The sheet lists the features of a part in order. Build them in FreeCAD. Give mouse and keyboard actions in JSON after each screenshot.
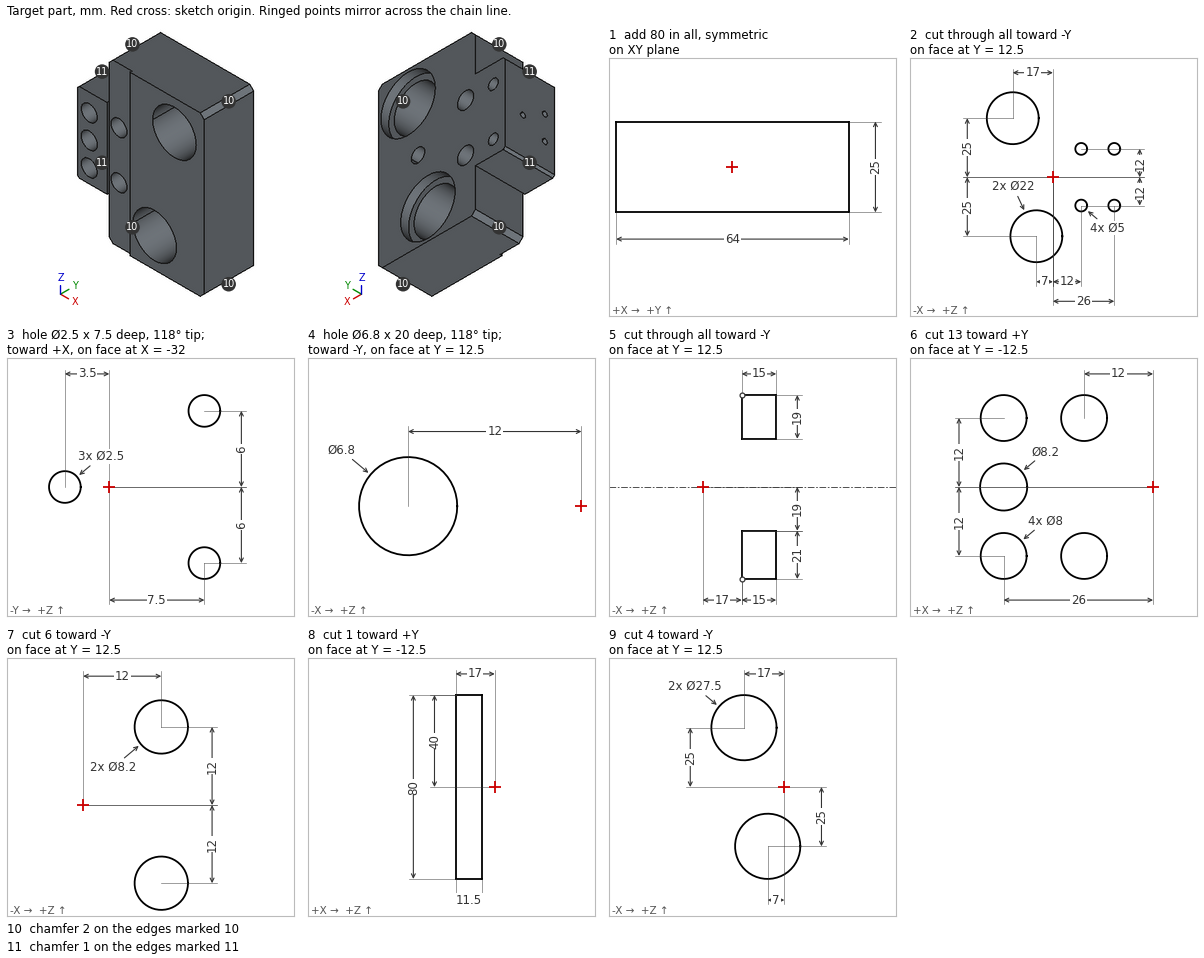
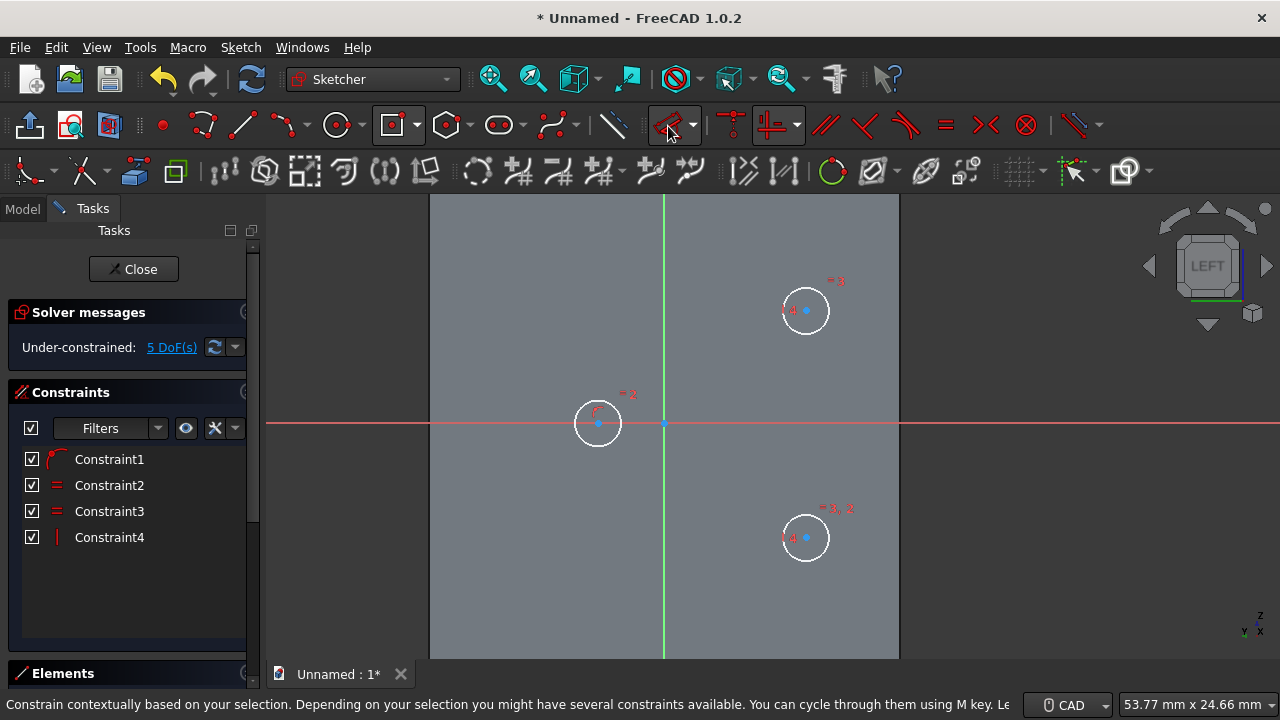
{"action": "left_click", "coordinate": [614, 407]}
{"action": "left_click", "coordinate": [636, 384]}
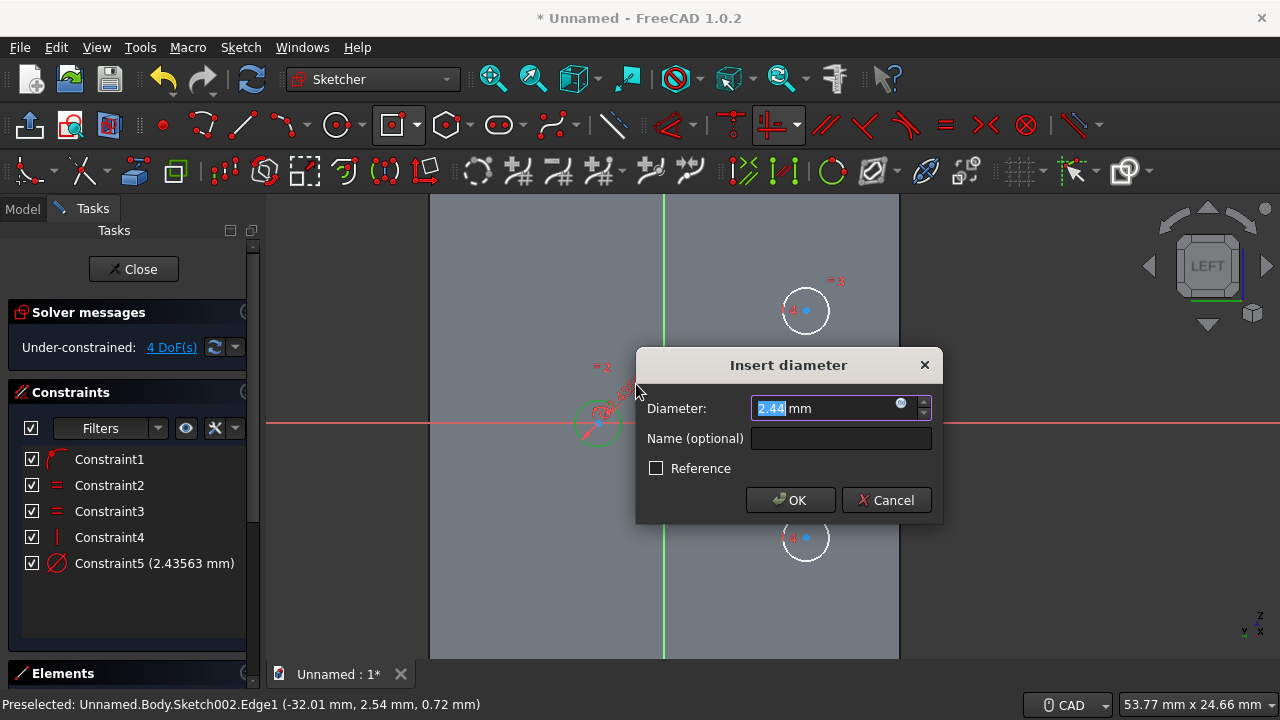
{"action": "type", "text": "2.5"}
{"action": "key", "text": "Return"}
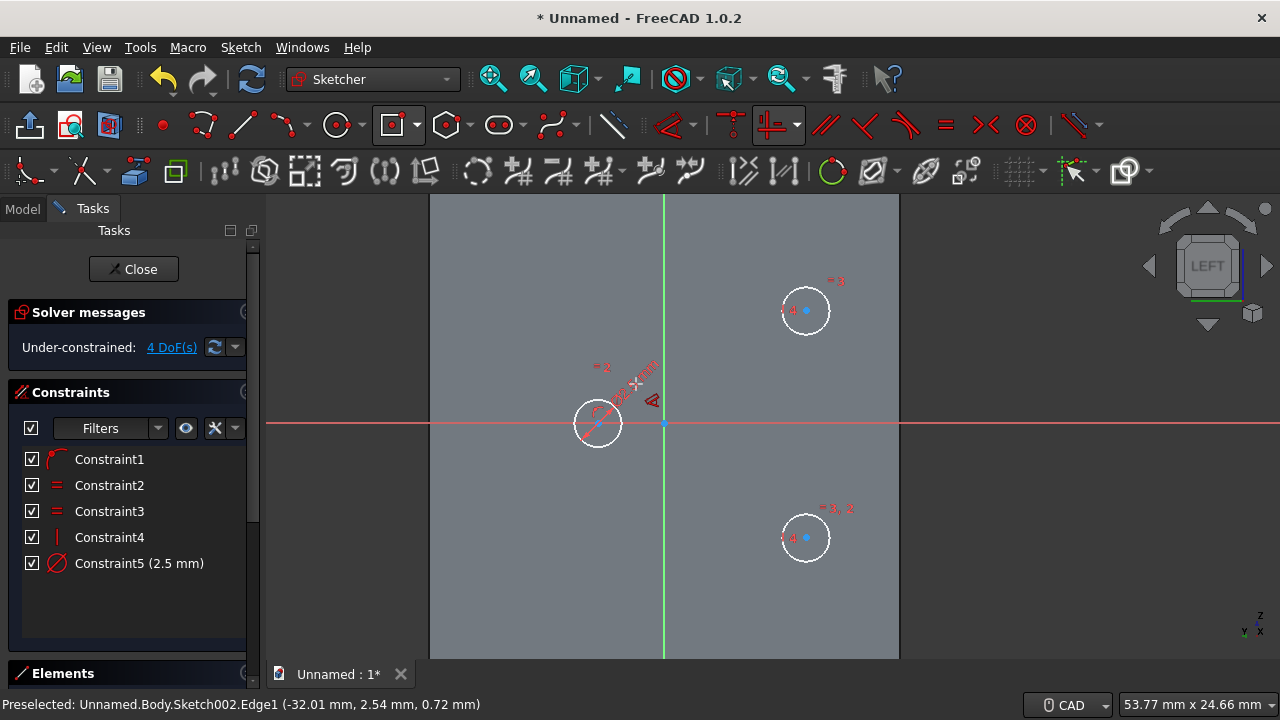
{"action": "left_click", "coordinate": [806, 538]}
{"action": "left_click", "coordinate": [840, 481]}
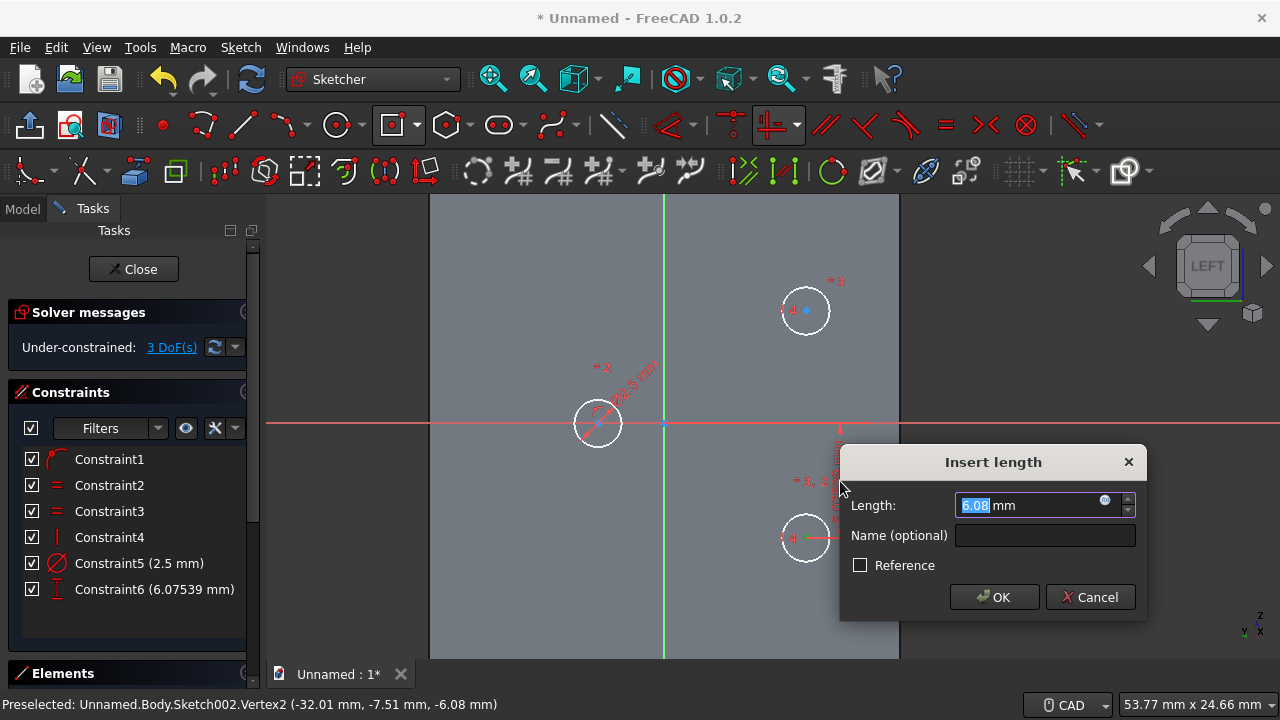
{"action": "type", "text": "6"}
{"action": "key", "text": "Return"}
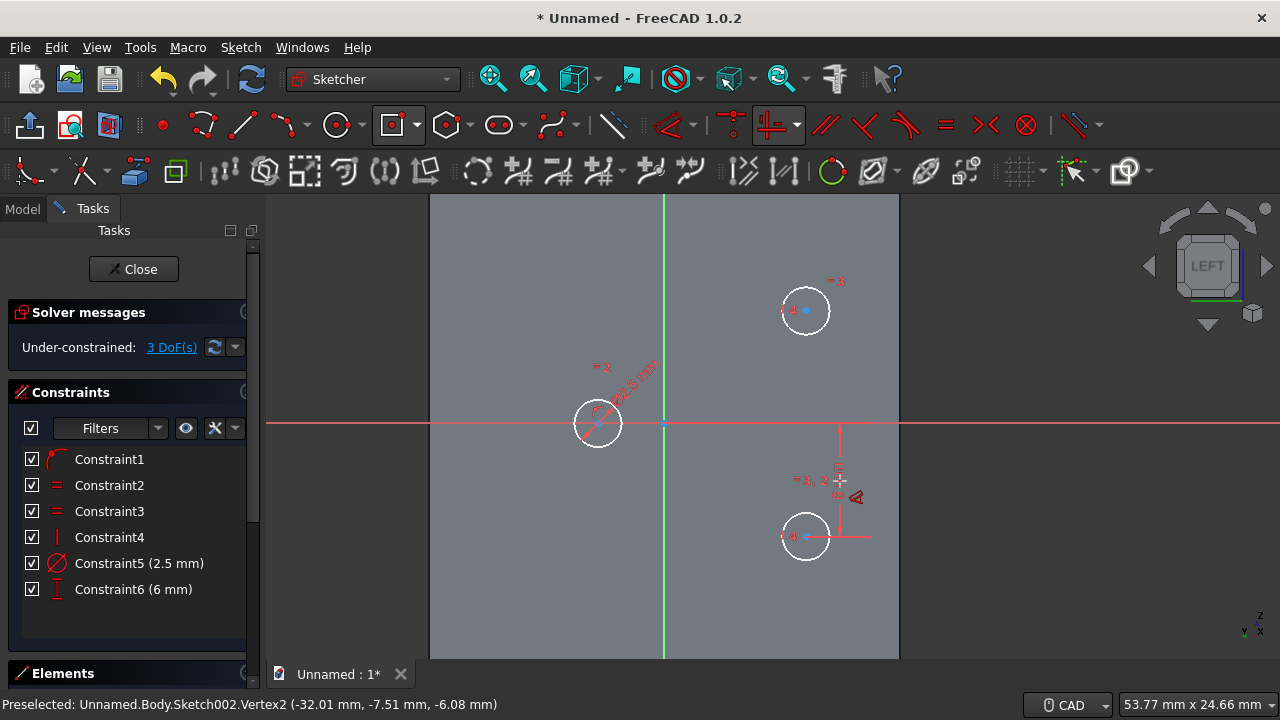
{"action": "left_click", "coordinate": [806, 311]}
{"action": "left_click", "coordinate": [840, 367]}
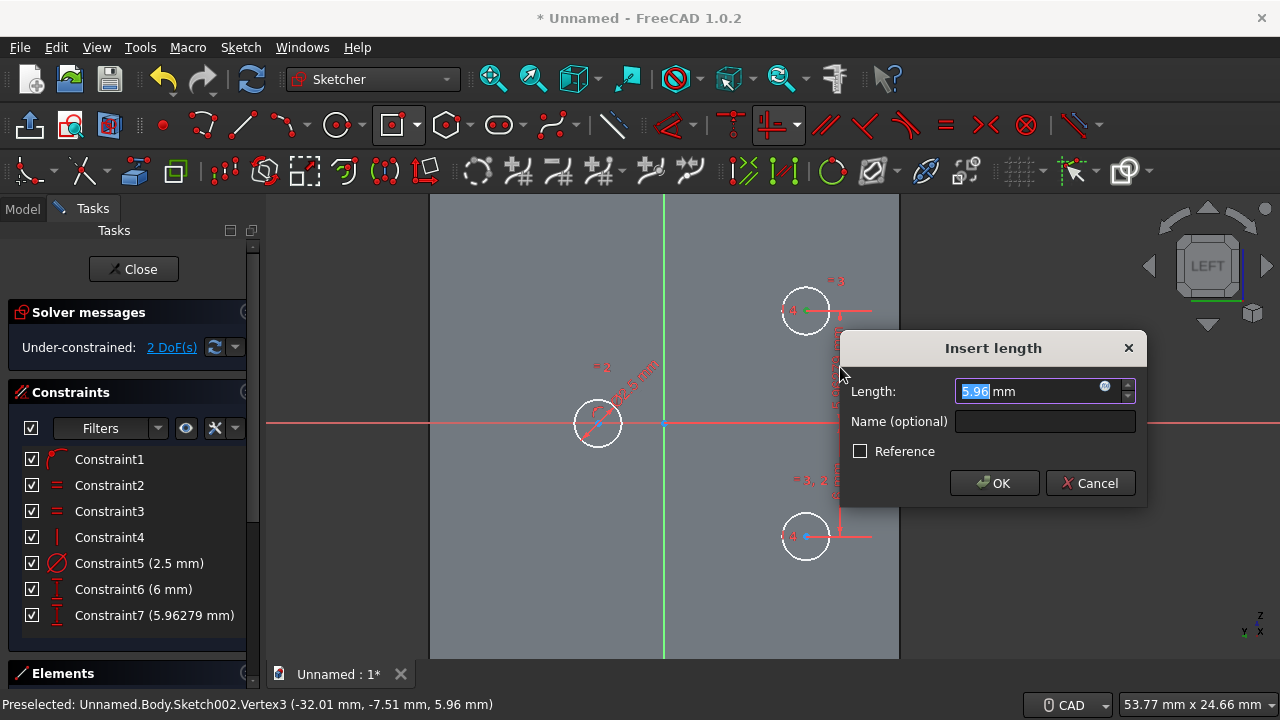
{"action": "type", "text": "6"}
{"action": "key", "text": "Return"}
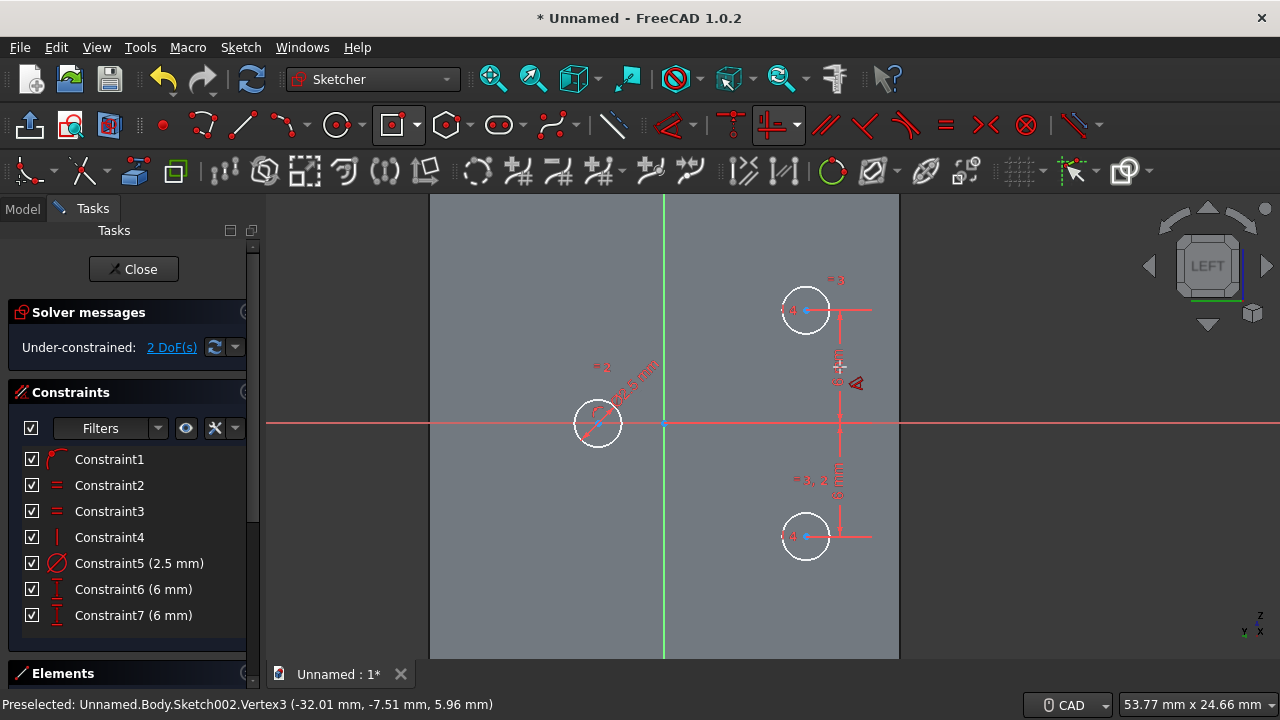
{"action": "left_click", "coordinate": [598, 423]}
{"action": "left_click", "coordinate": [631, 457]}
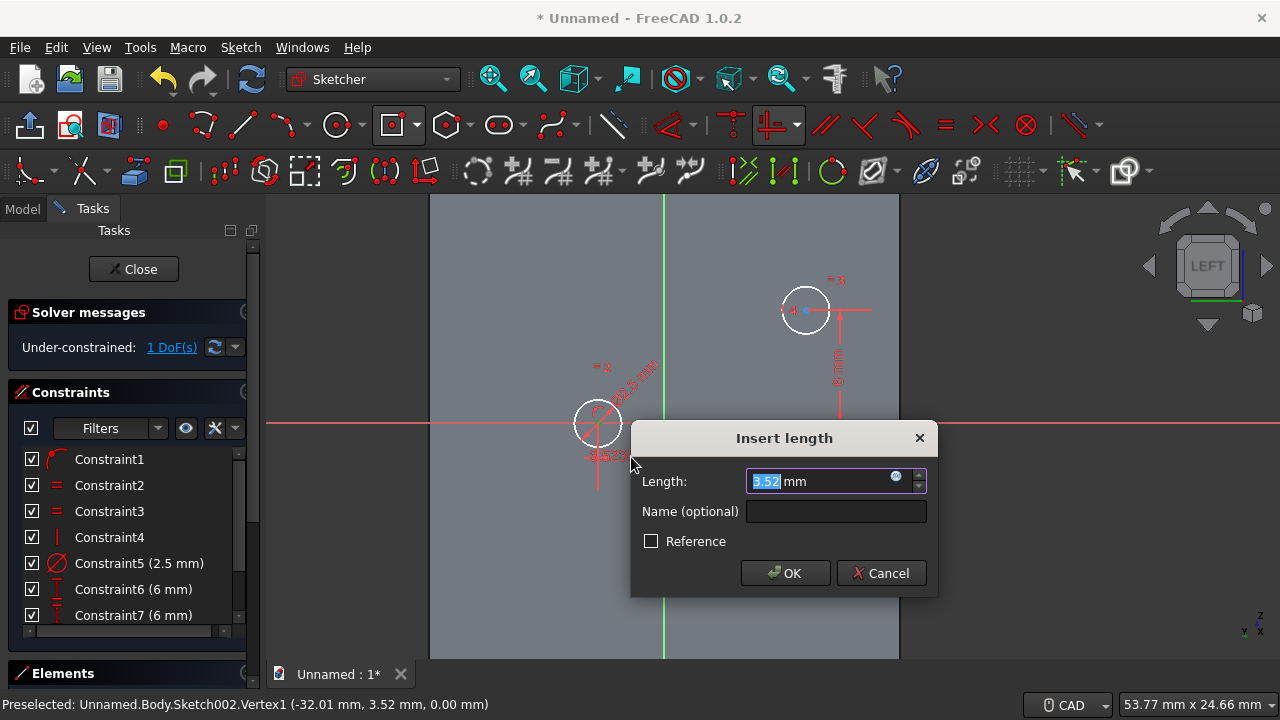
{"action": "type", "text": "3.5"}
{"action": "key", "text": "Return"}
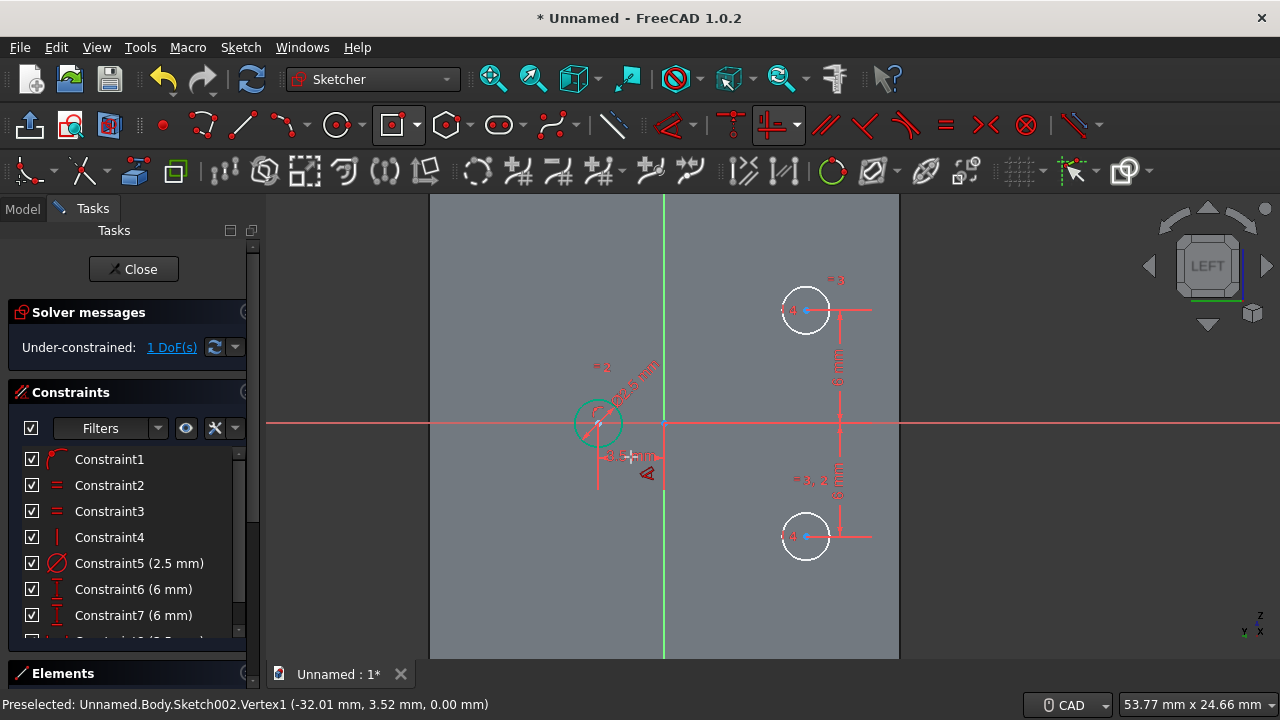
{"action": "left_click", "coordinate": [806, 537]}
{"action": "left_click", "coordinate": [735, 571]}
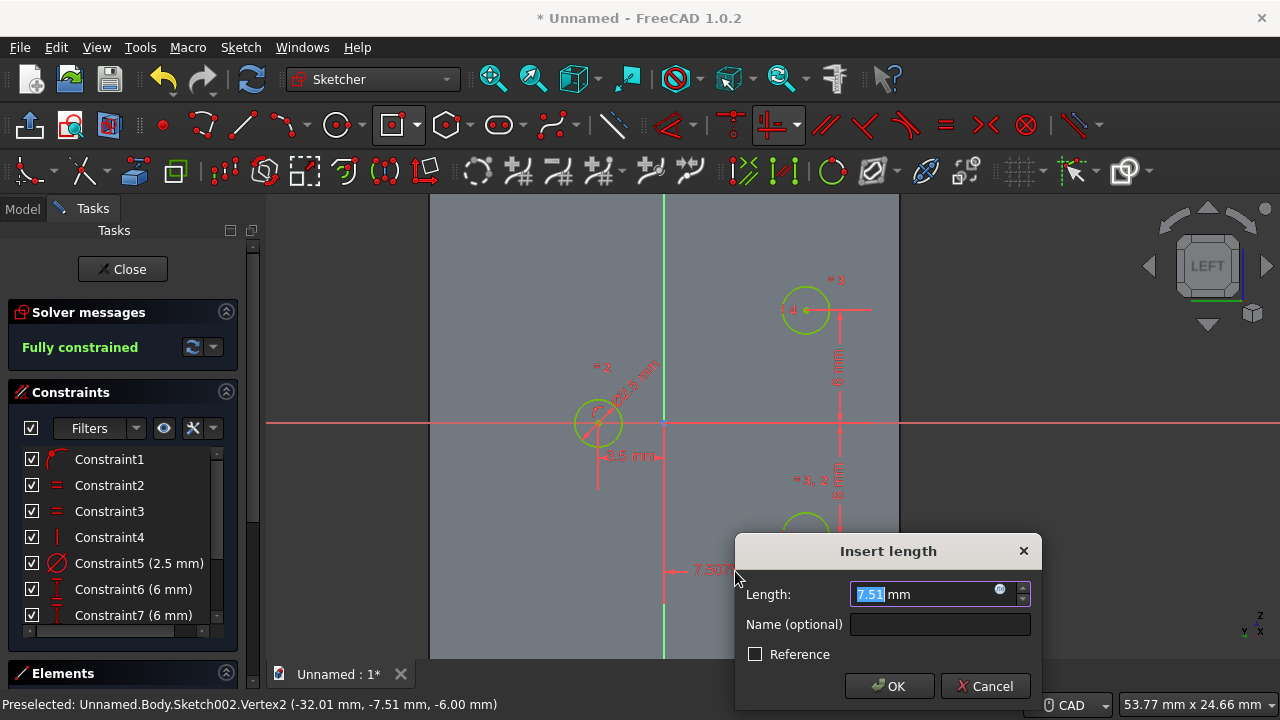
{"action": "type", "text": "7.5"}
{"action": "key", "text": "Return"}
{"action": "key", "text": "Escape"}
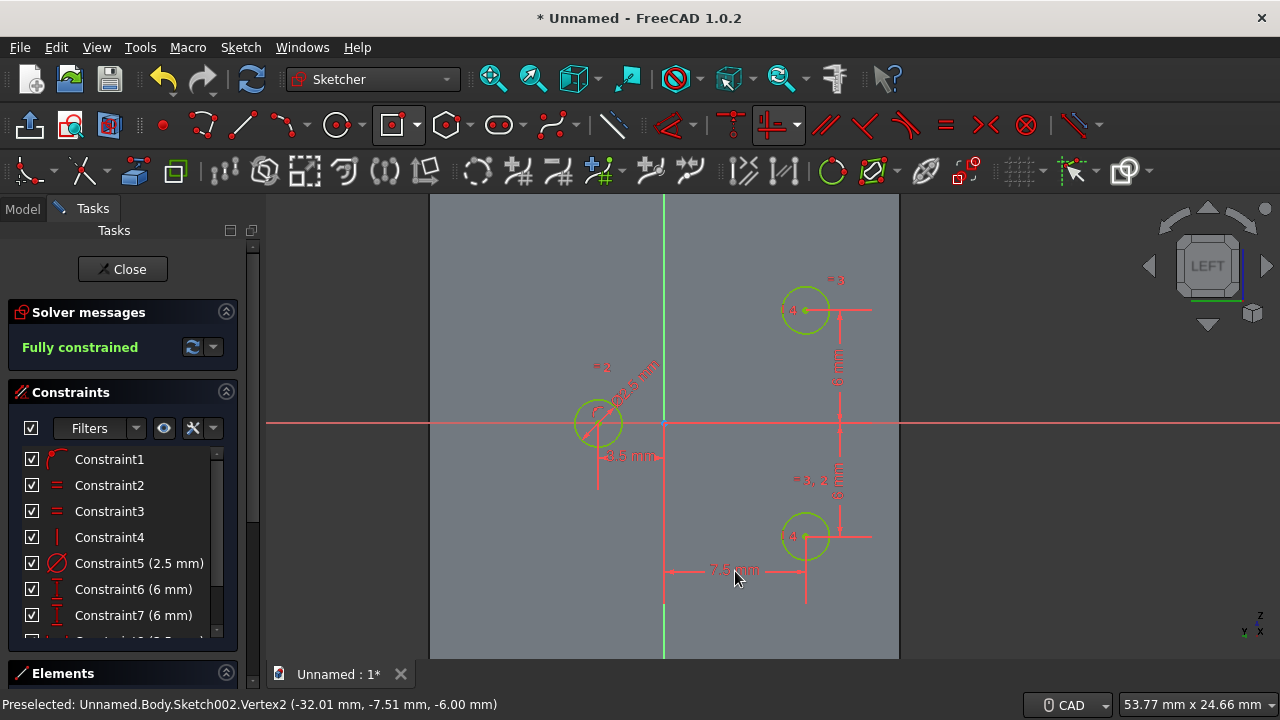
{"action": "left_click", "coordinate": [123, 269]}